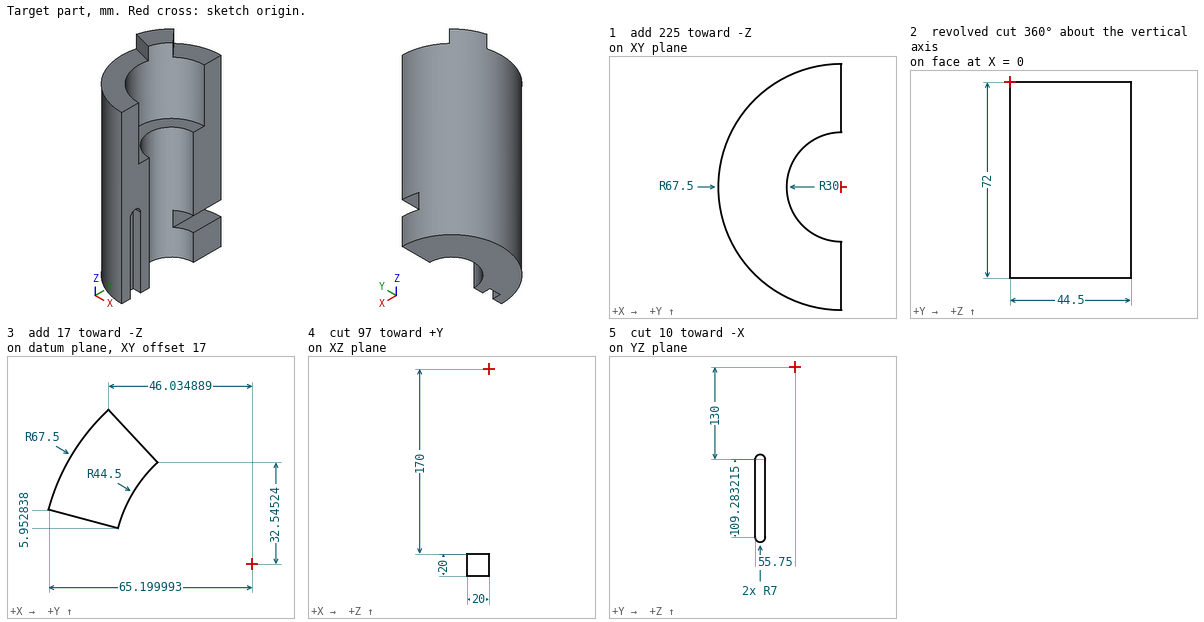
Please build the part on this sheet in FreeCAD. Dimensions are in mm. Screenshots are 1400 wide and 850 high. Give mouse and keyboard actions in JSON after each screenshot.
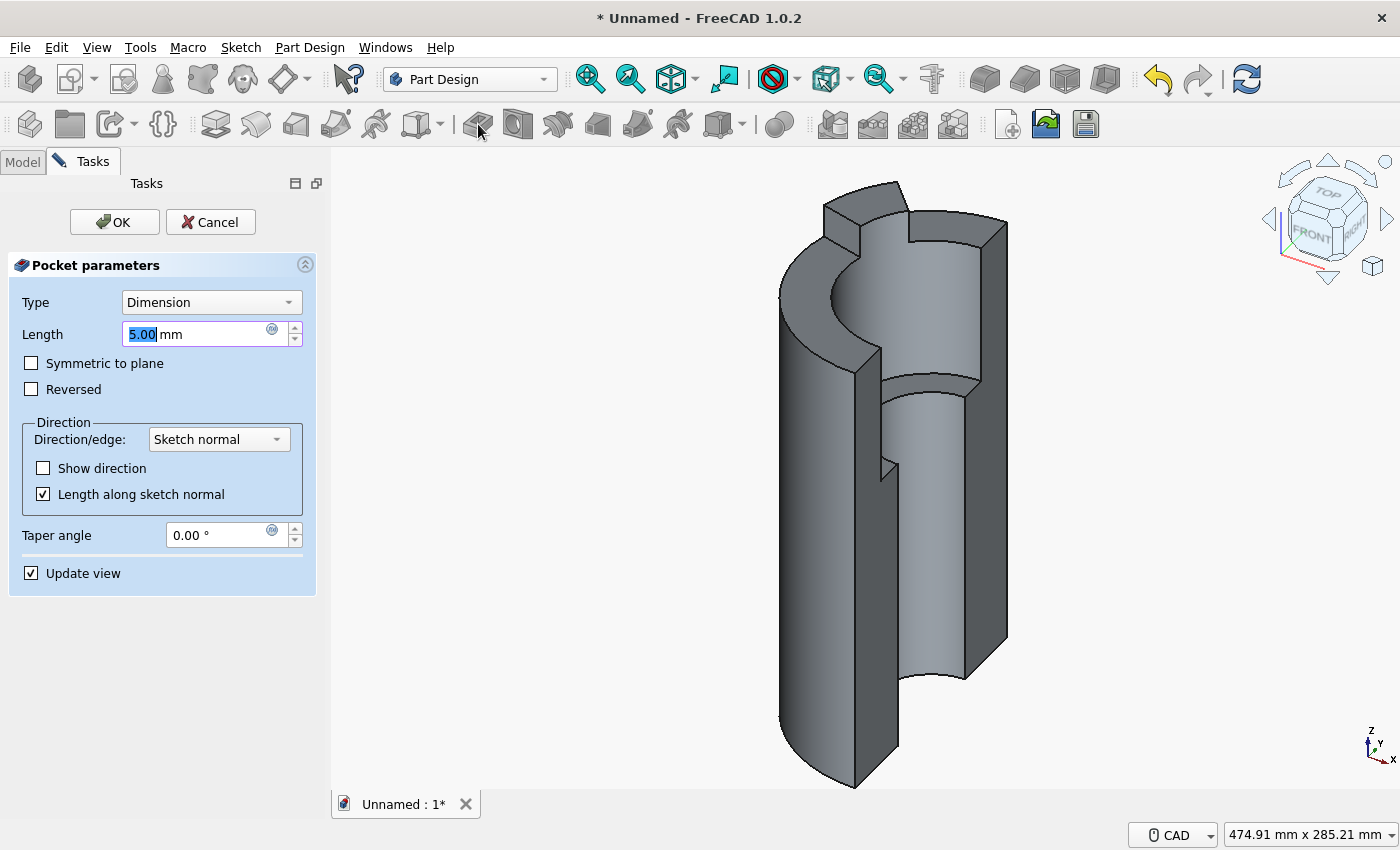
{"action": "type", "text": "97"}
{"action": "key", "text": "Tab"}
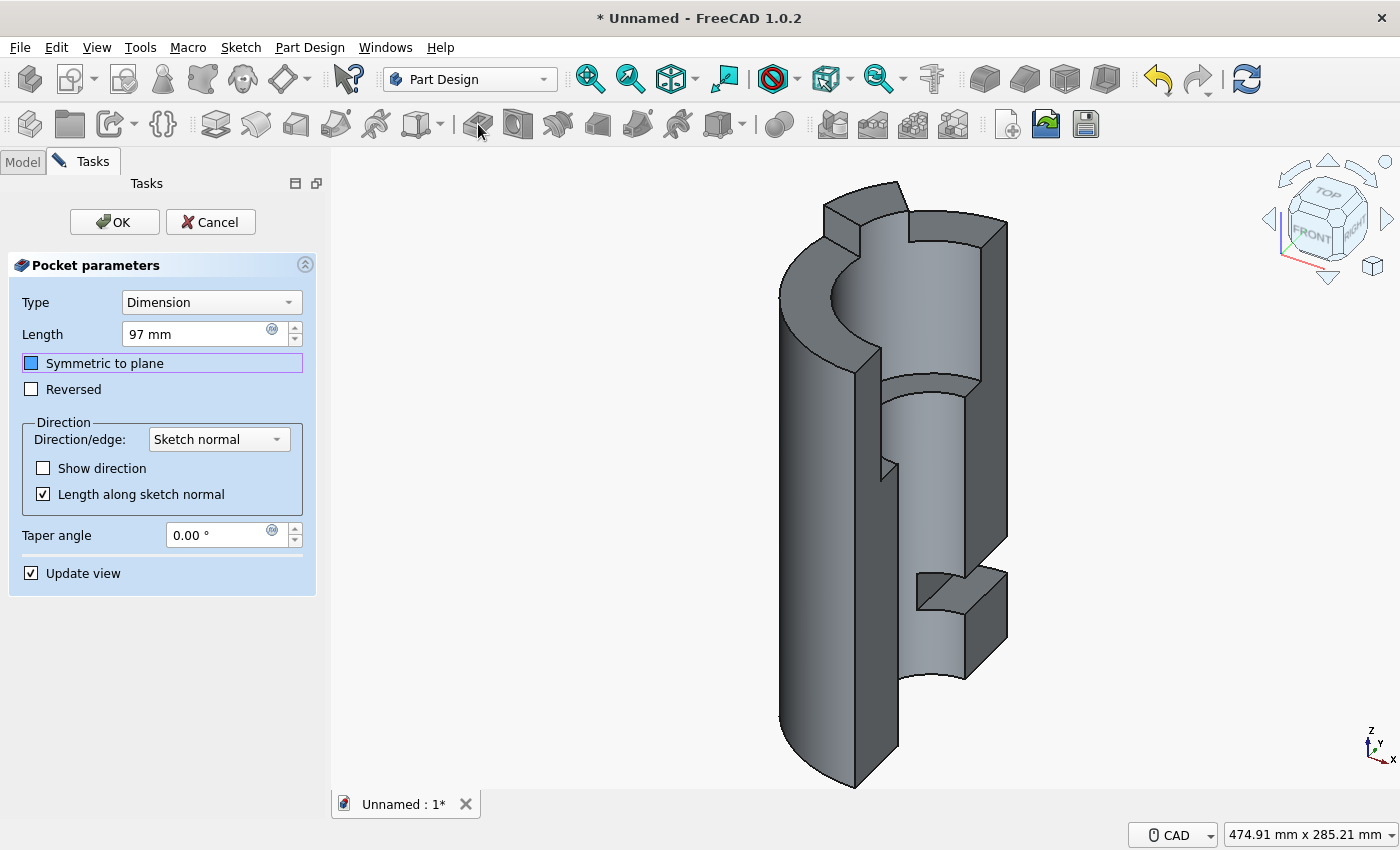
{"action": "left_click", "coordinate": [115, 222]}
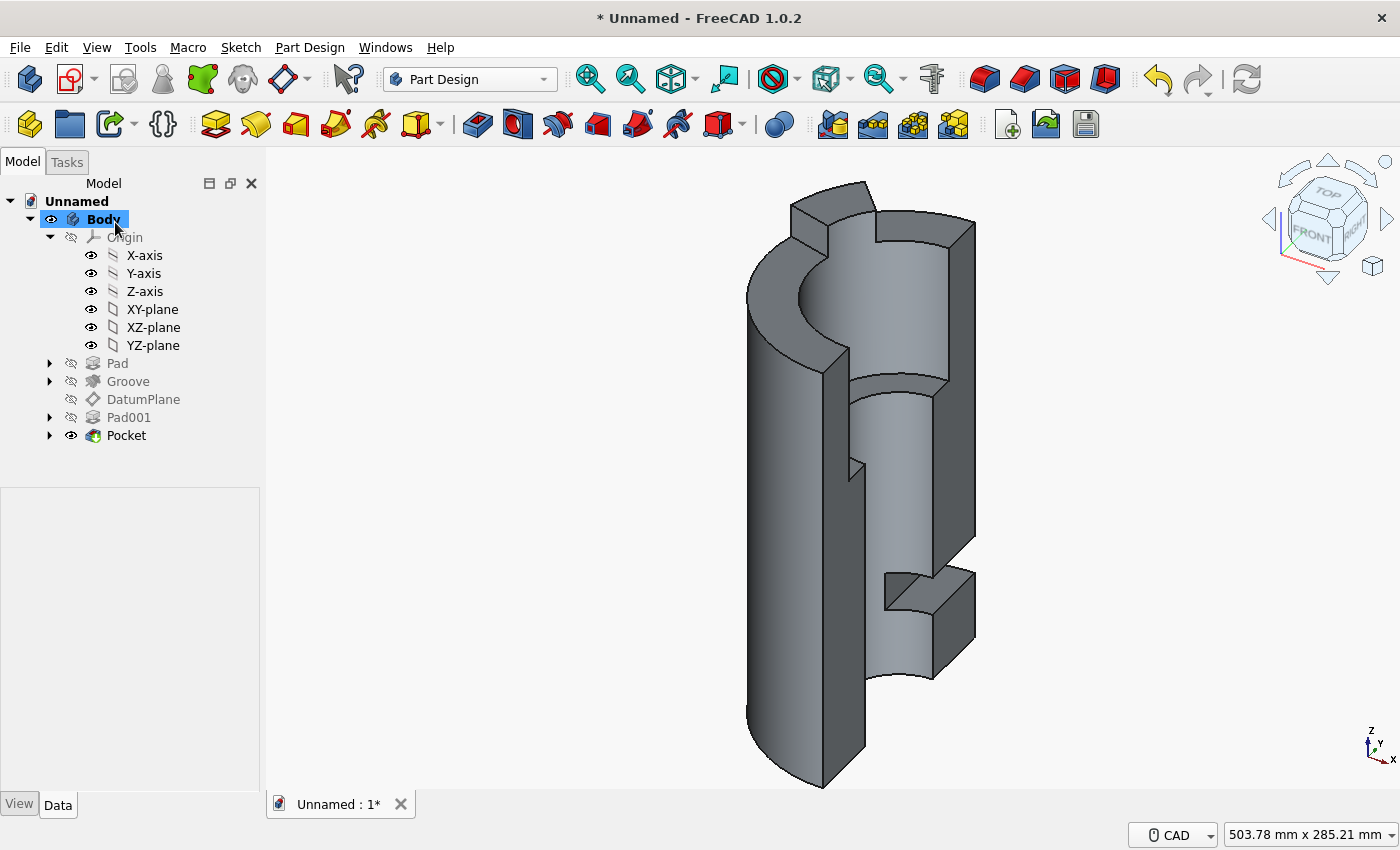
{"action": "left_click", "coordinate": [70, 80]}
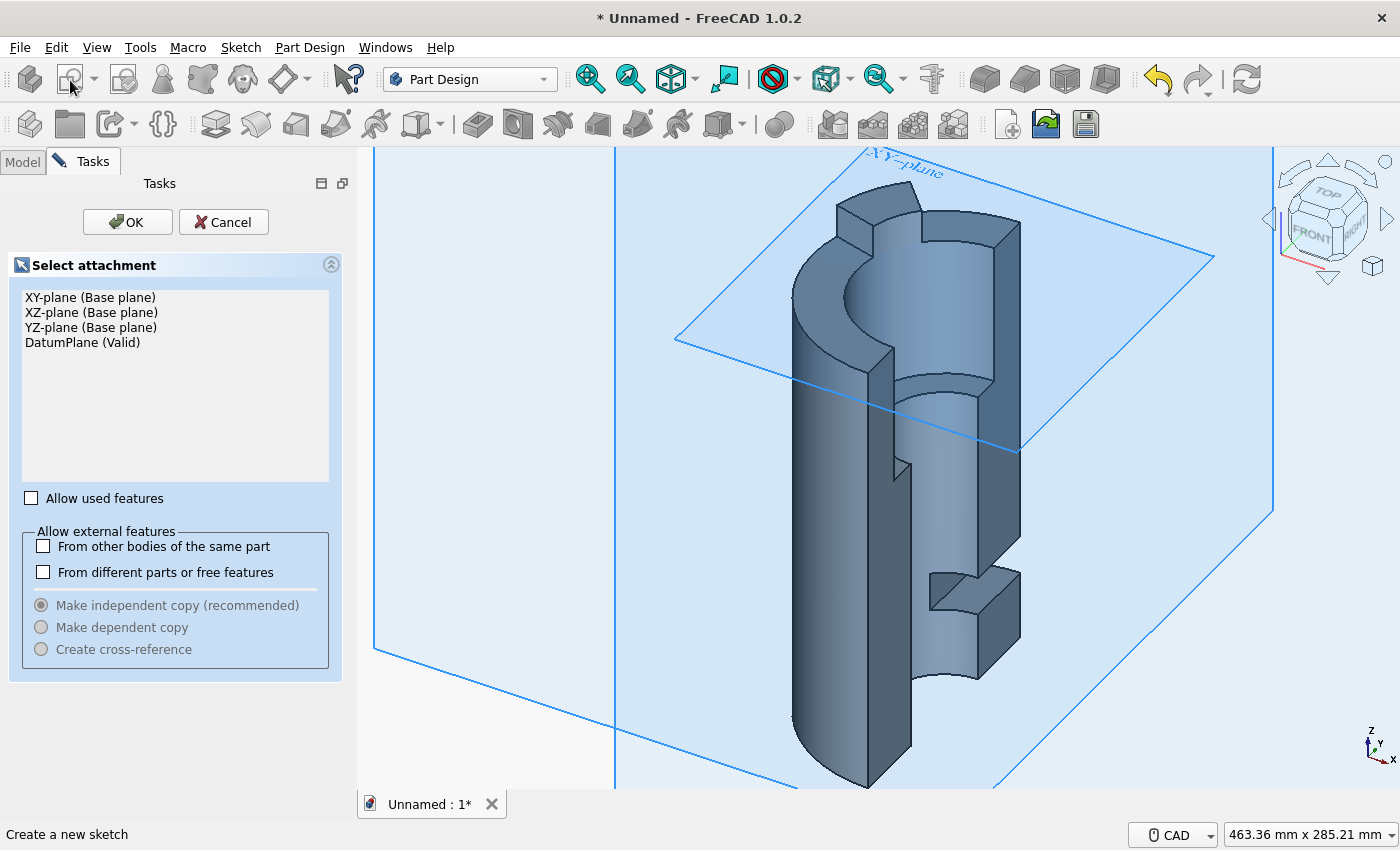
{"action": "left_click", "coordinate": [82, 328]}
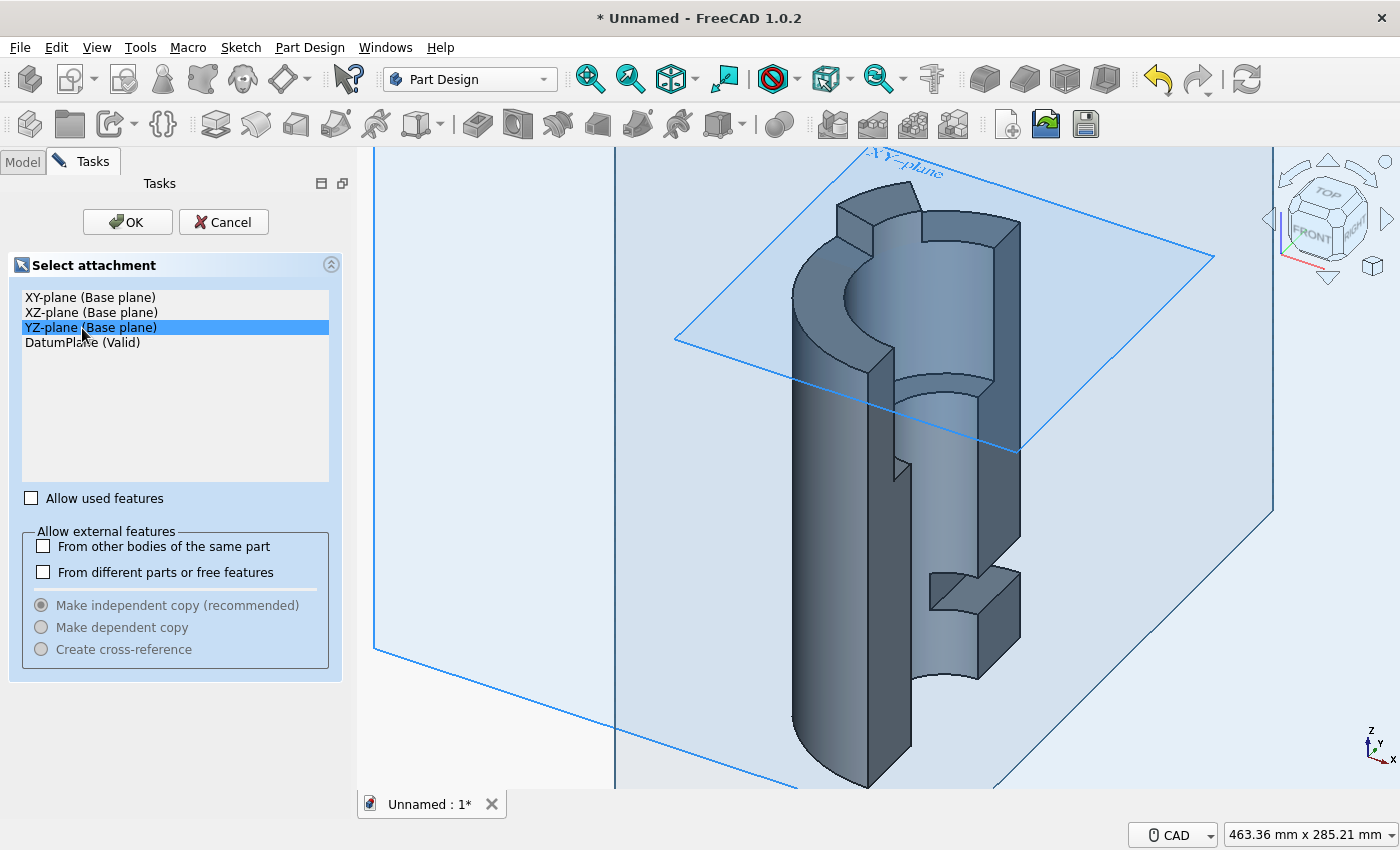
{"action": "left_click", "coordinate": [128, 222]}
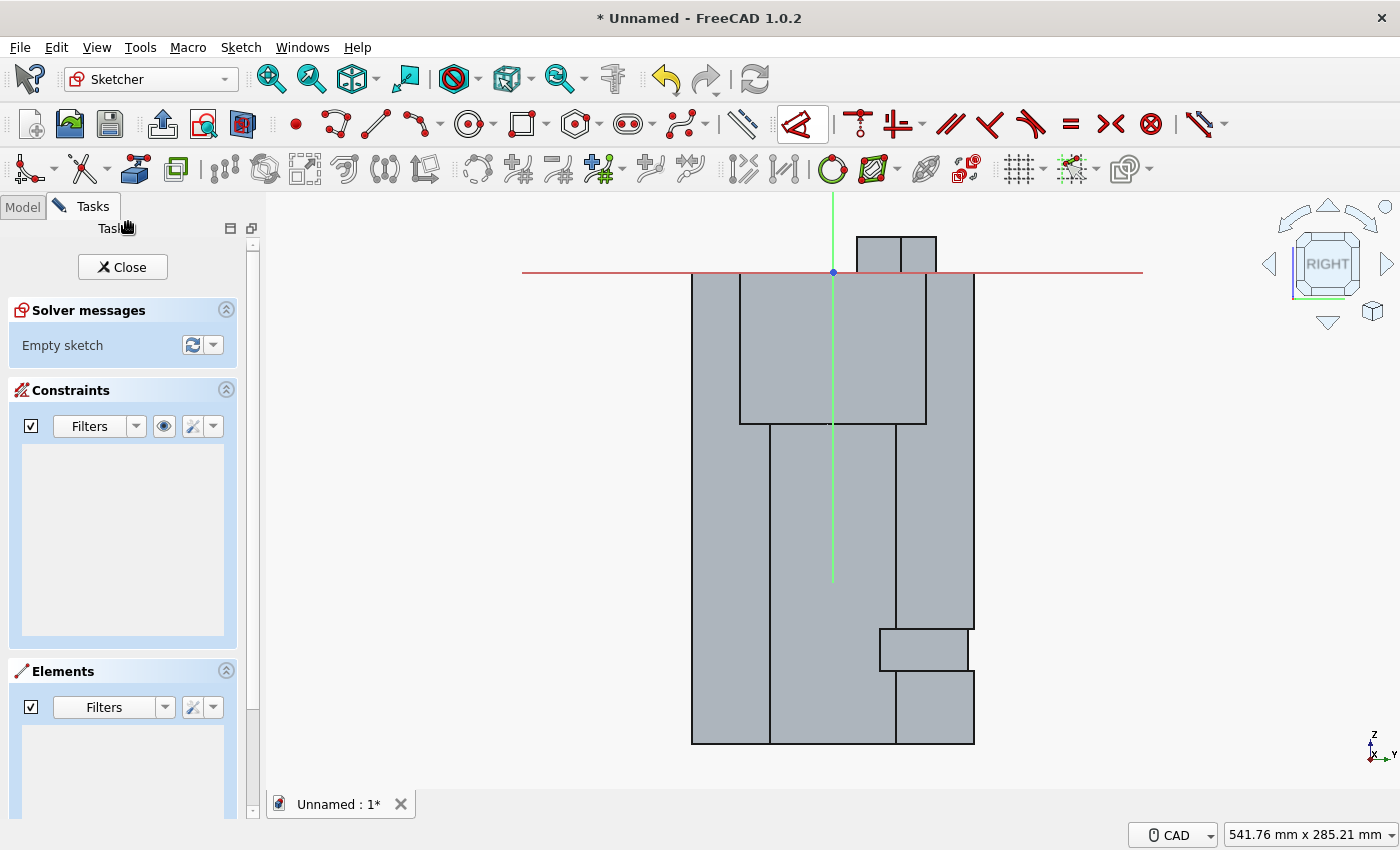
{"action": "scroll", "coordinate": [744, 409], "scroll_direction": "down", "scroll_amount": 2}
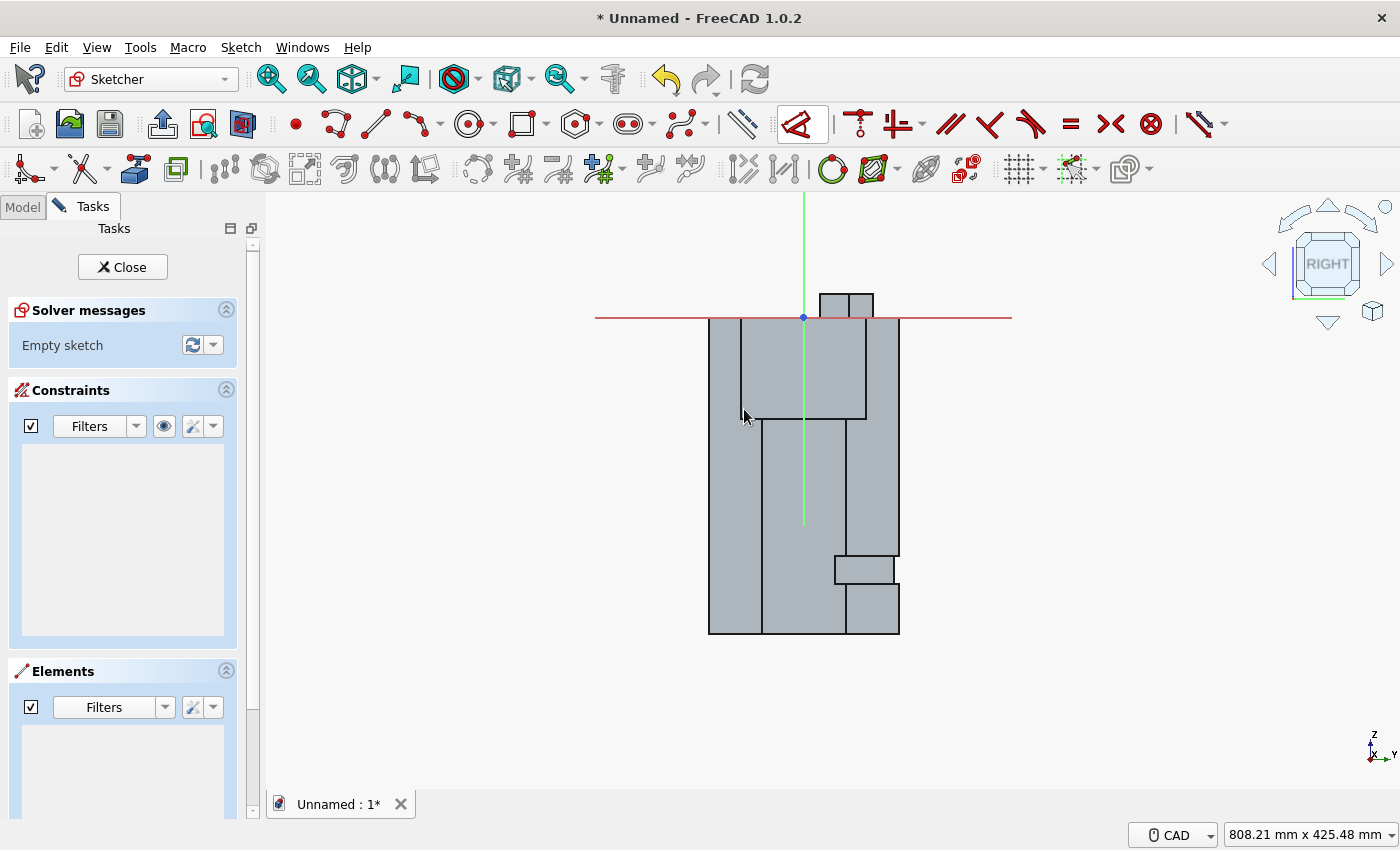
{"action": "key", "text": "g s"}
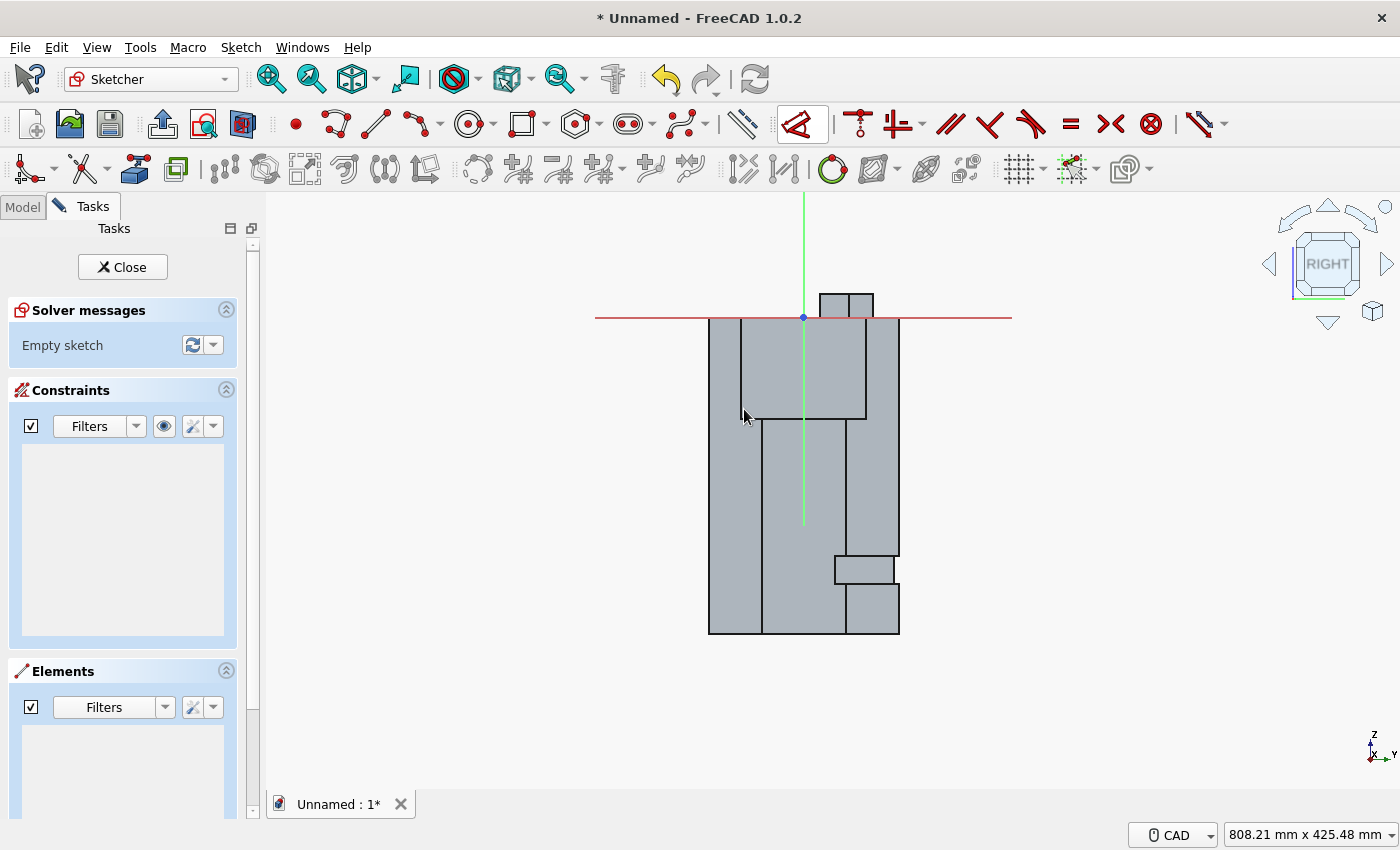
{"action": "scroll", "coordinate": [735, 654], "scroll_direction": "up", "scroll_amount": 5}